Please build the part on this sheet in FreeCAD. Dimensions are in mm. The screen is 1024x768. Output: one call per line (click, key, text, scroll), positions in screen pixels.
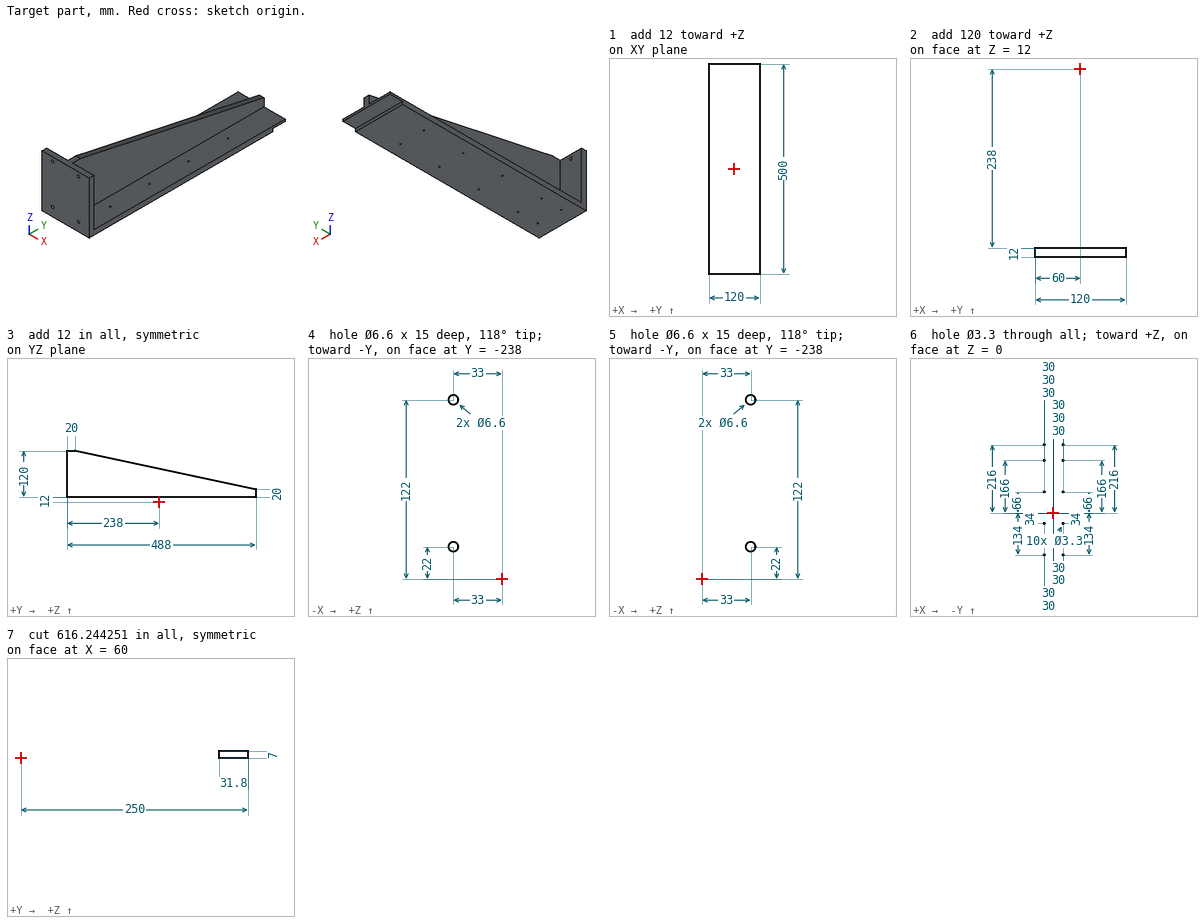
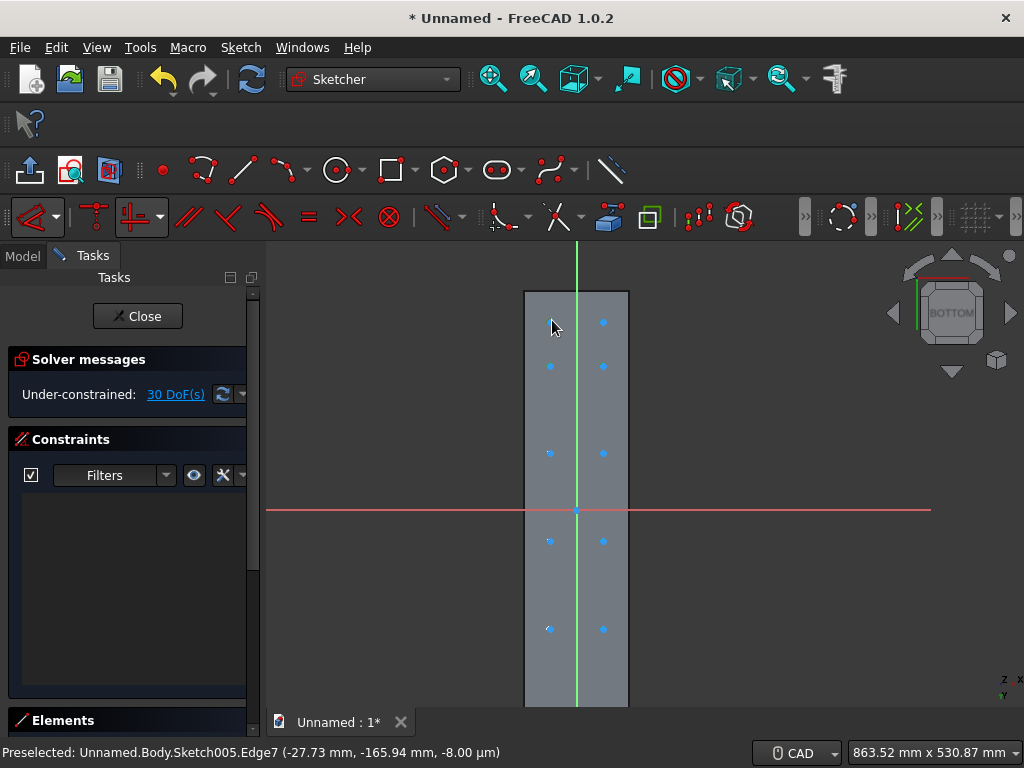
scroll(552, 451, up, 10)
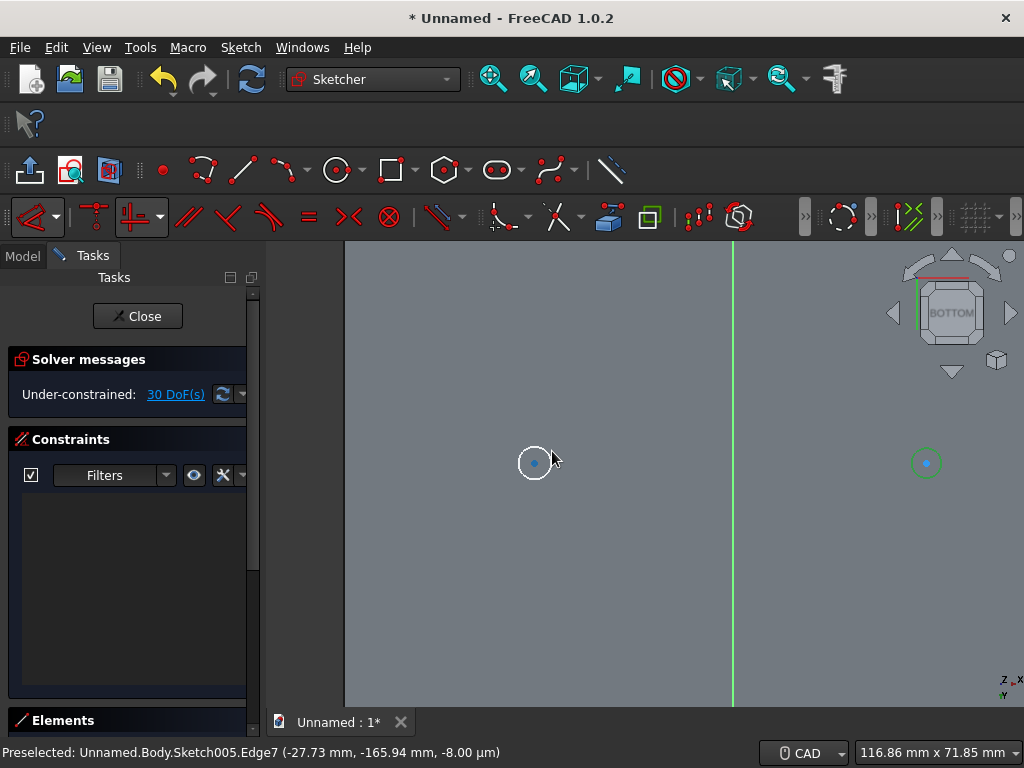
click(546, 452)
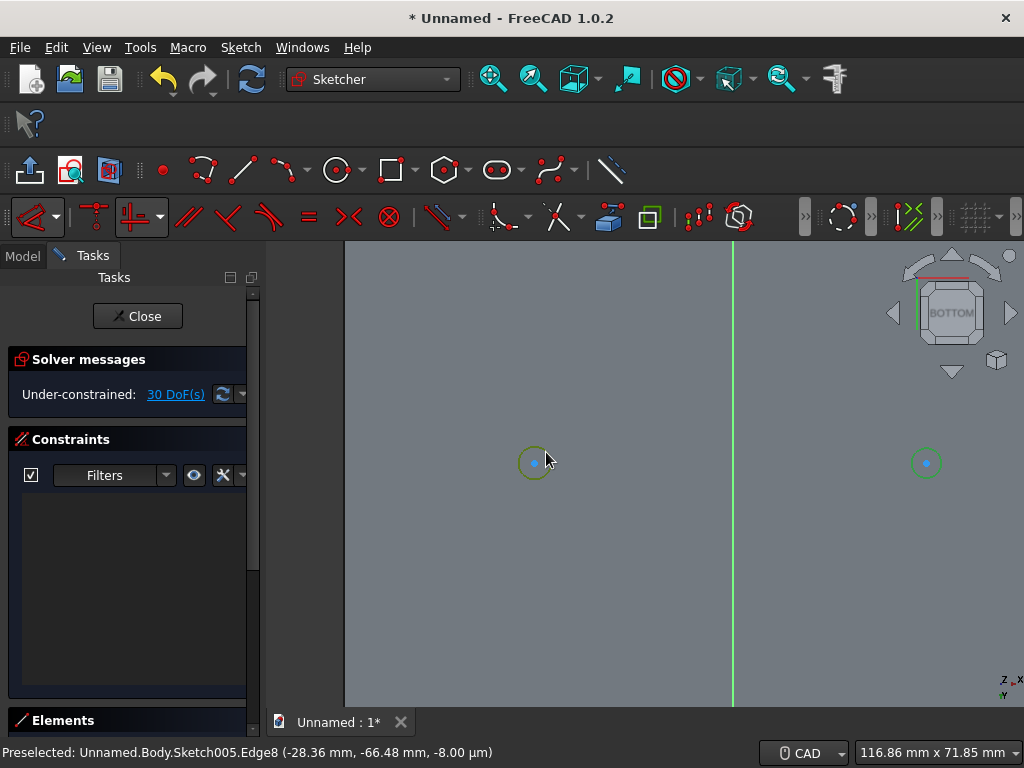
scroll(552, 451, down, 10)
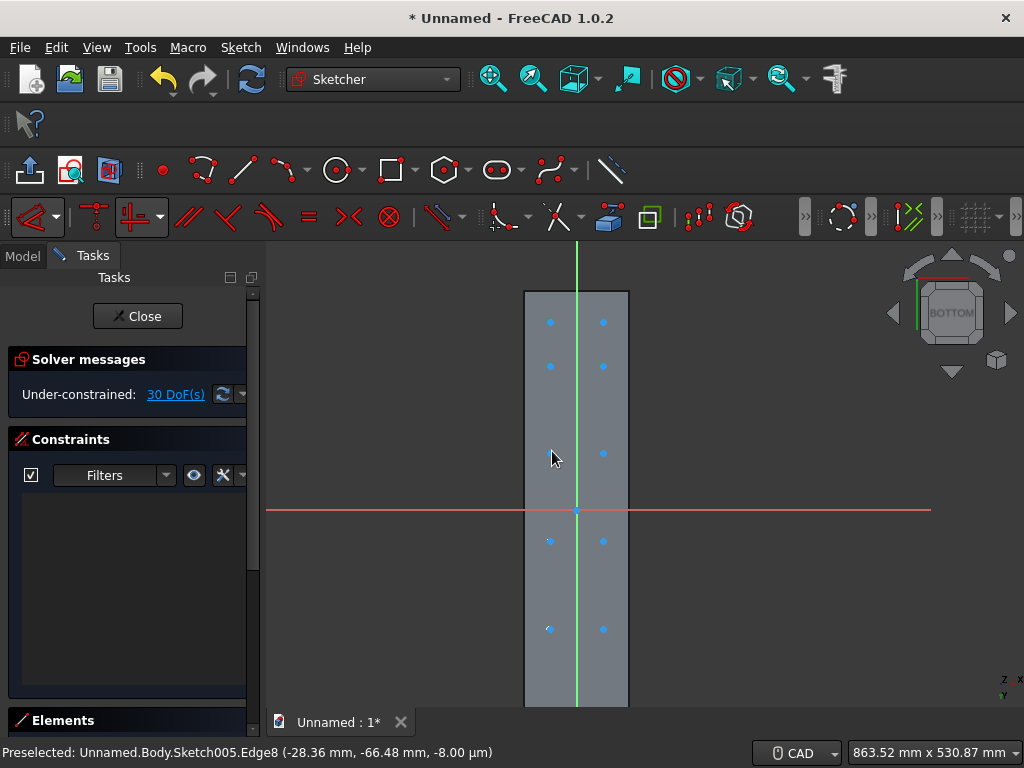
scroll(552, 539, up, 9)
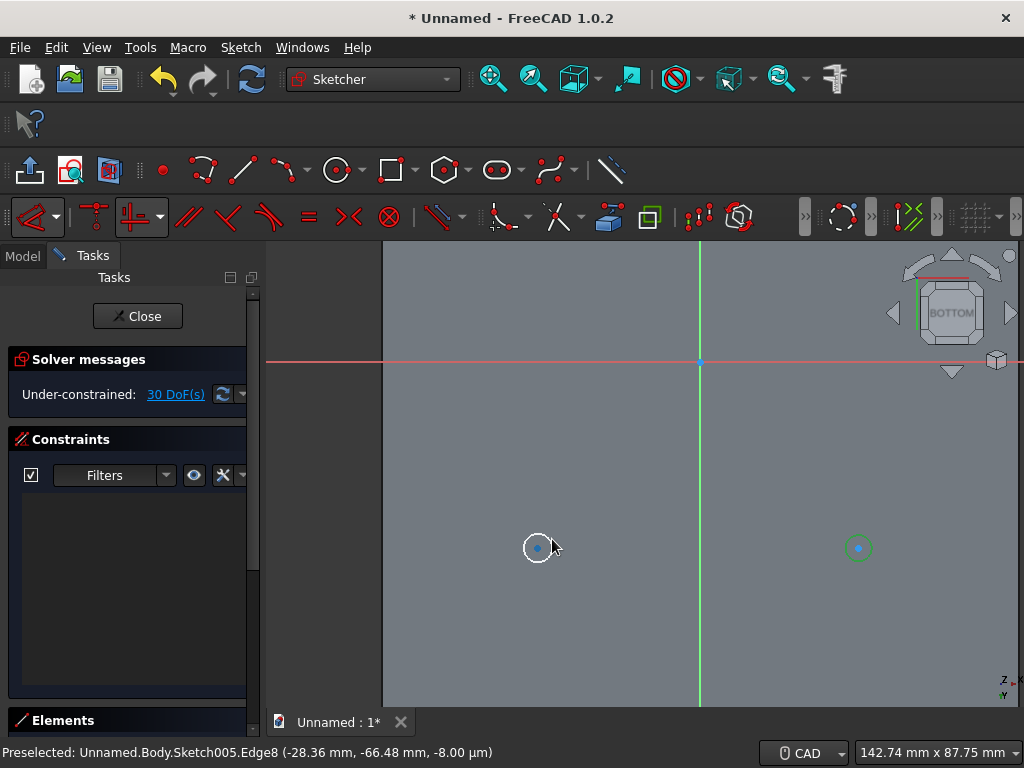
click(548, 538)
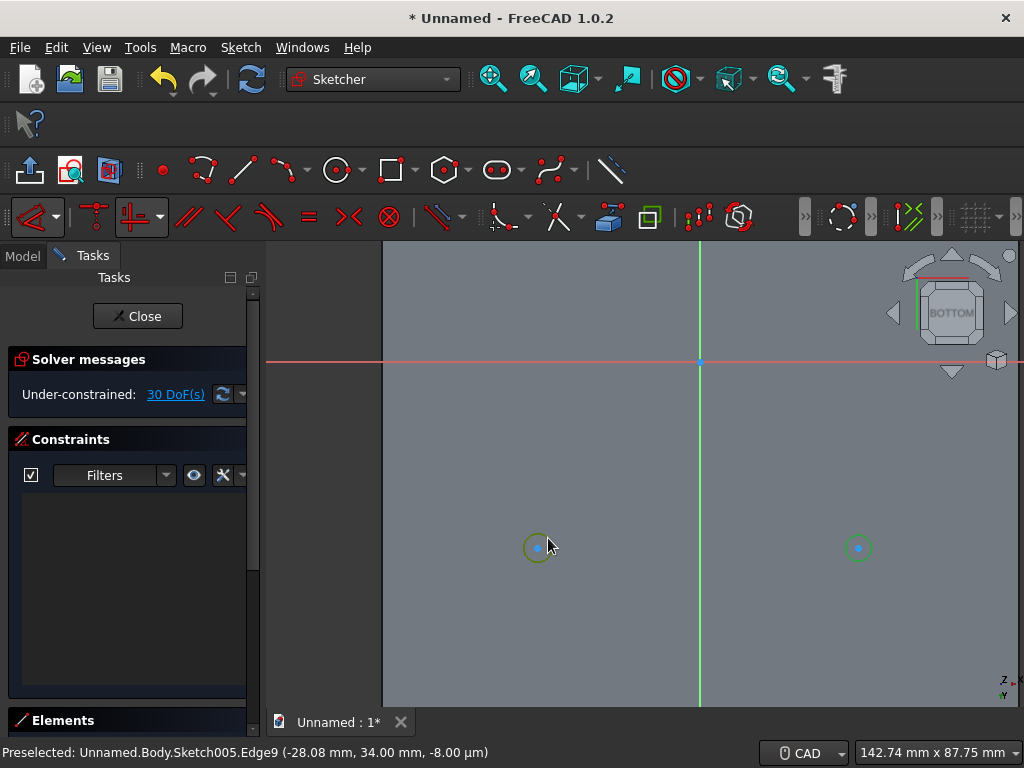
scroll(552, 539, down, 9)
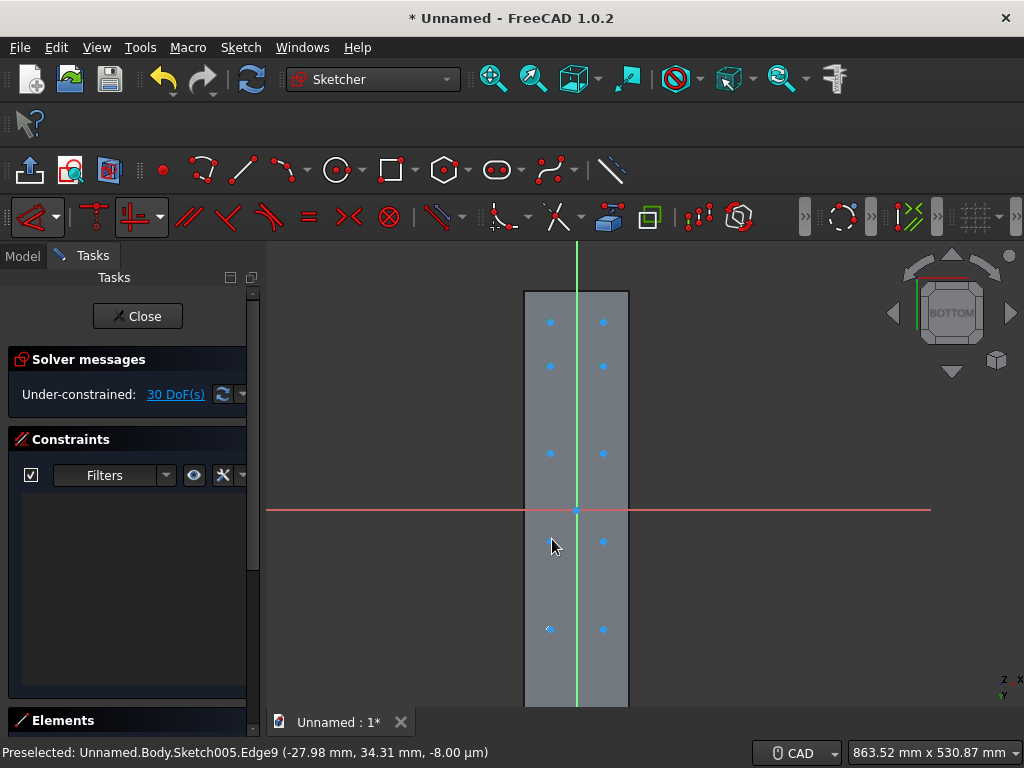
scroll(552, 627, up, 9)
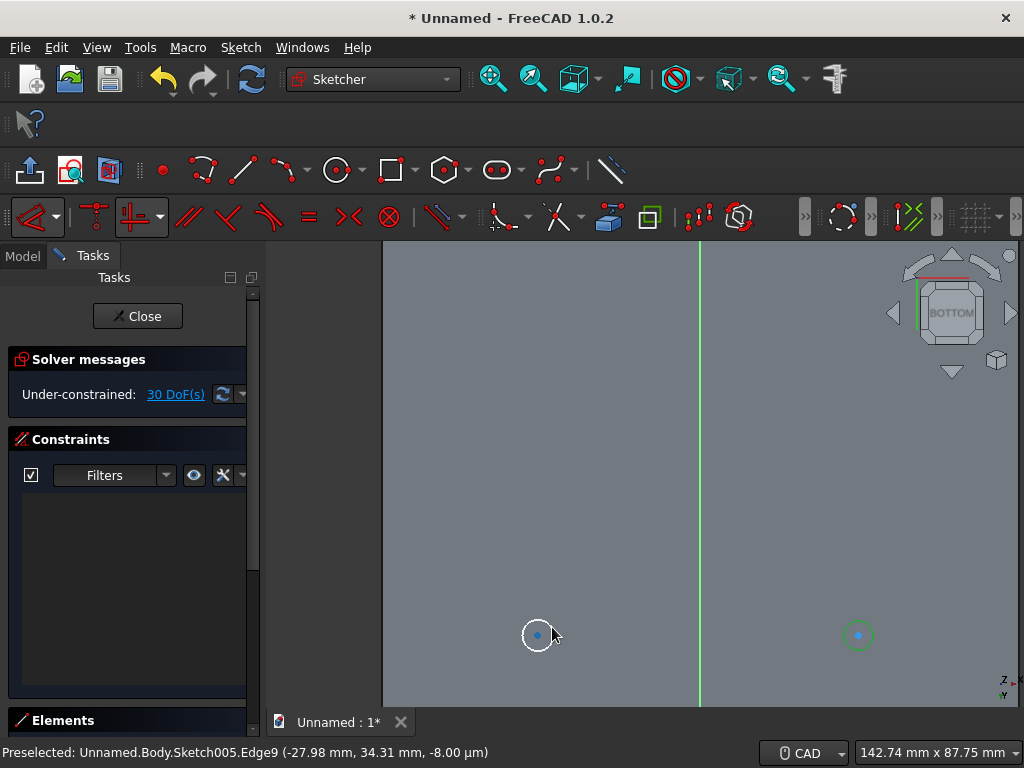
click(549, 624)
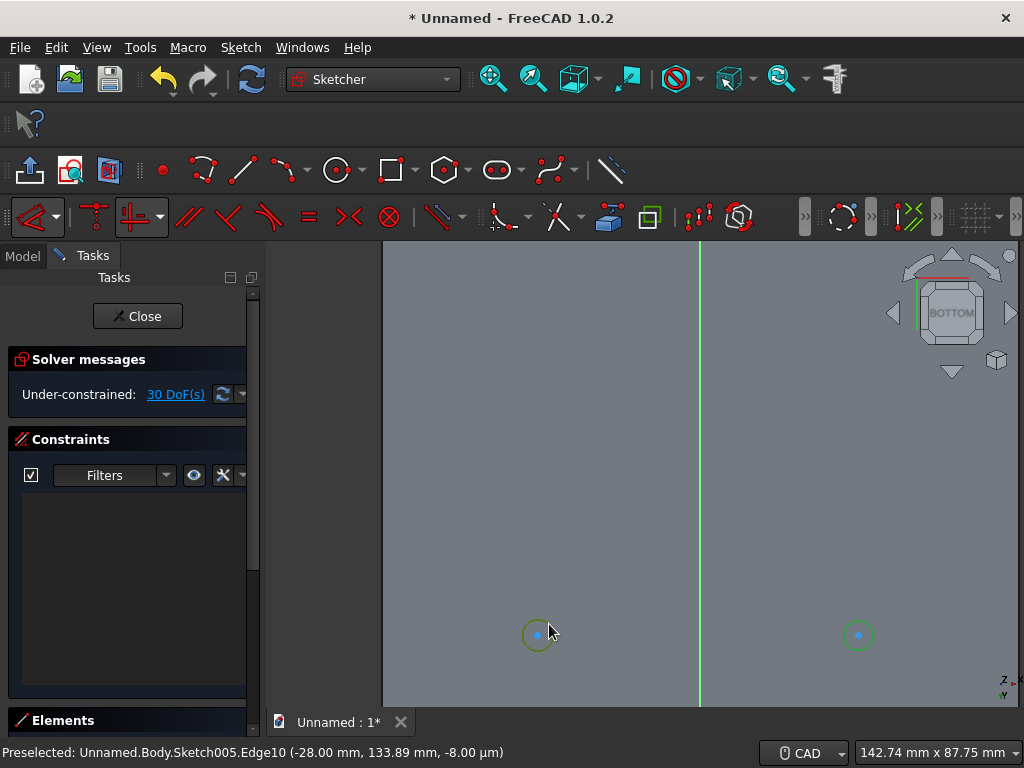
click(310, 218)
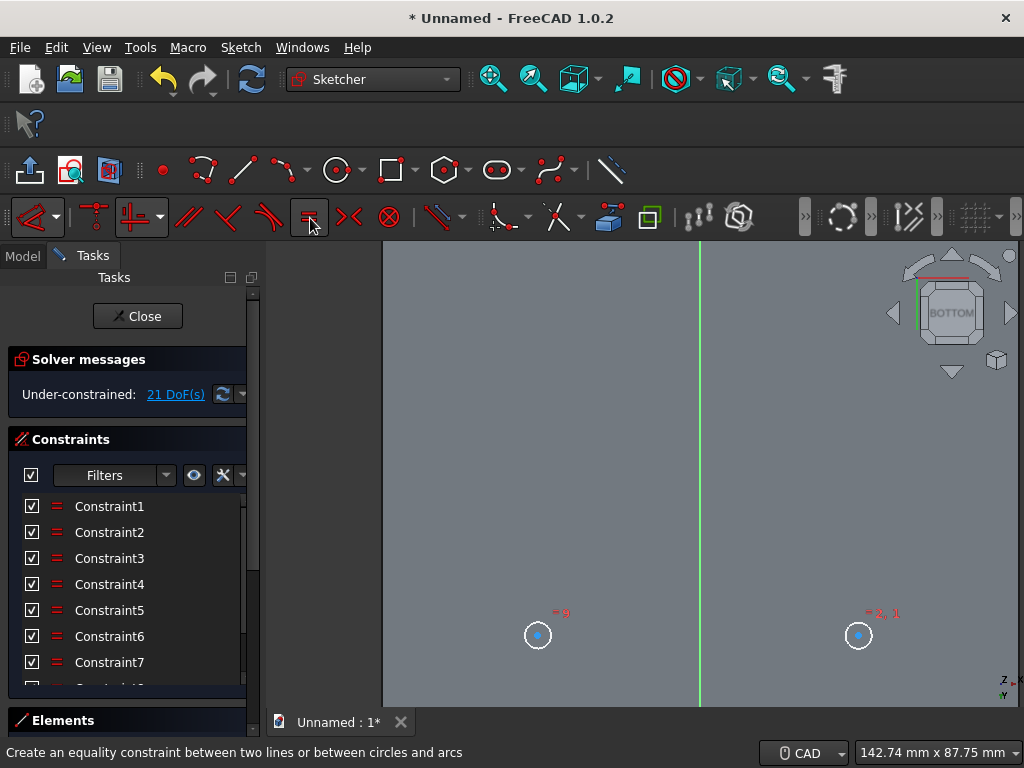
scroll(552, 627, down, 9)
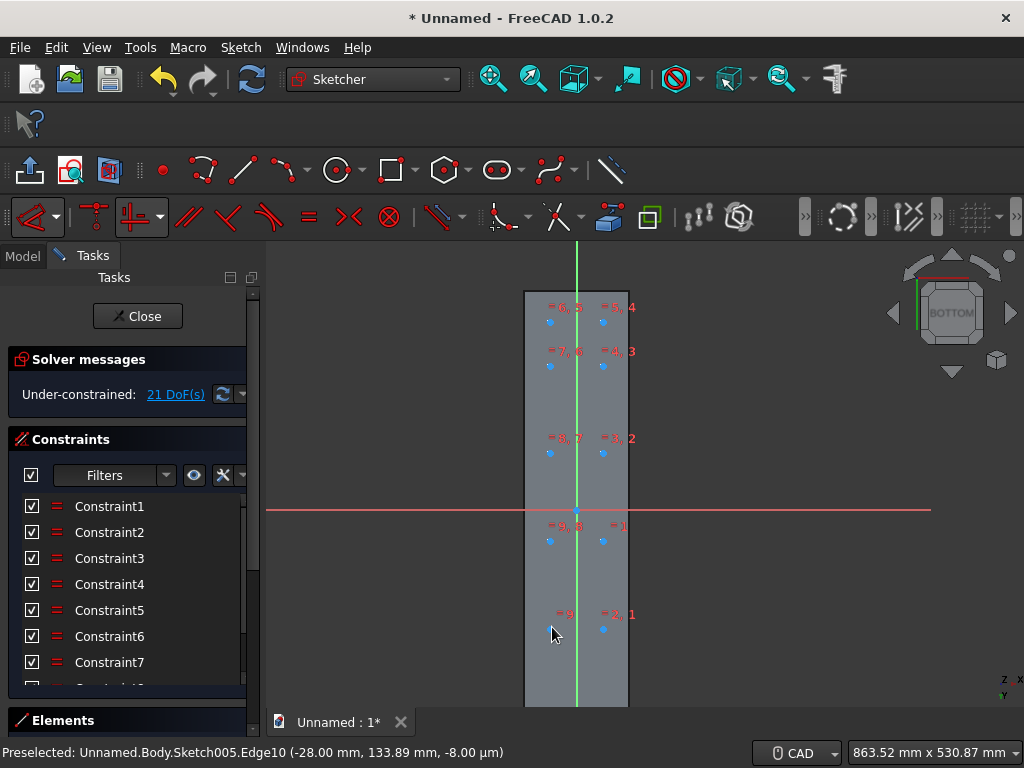
scroll(605, 540, up, 14)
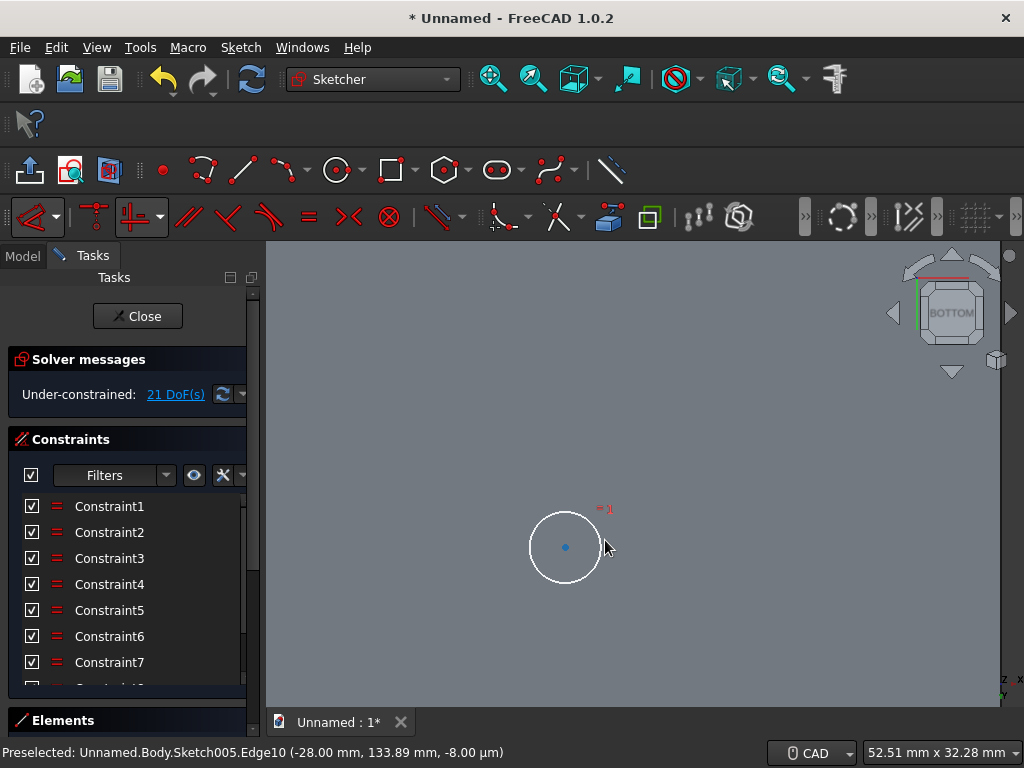
click(590, 522)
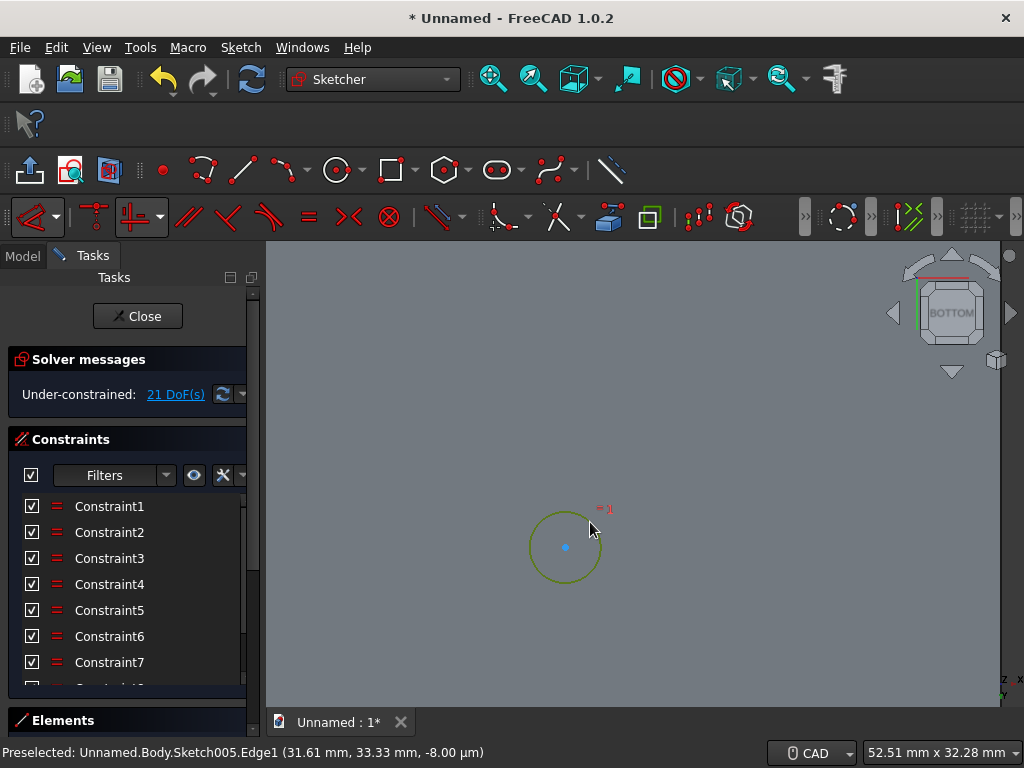
key(k)
key(o)